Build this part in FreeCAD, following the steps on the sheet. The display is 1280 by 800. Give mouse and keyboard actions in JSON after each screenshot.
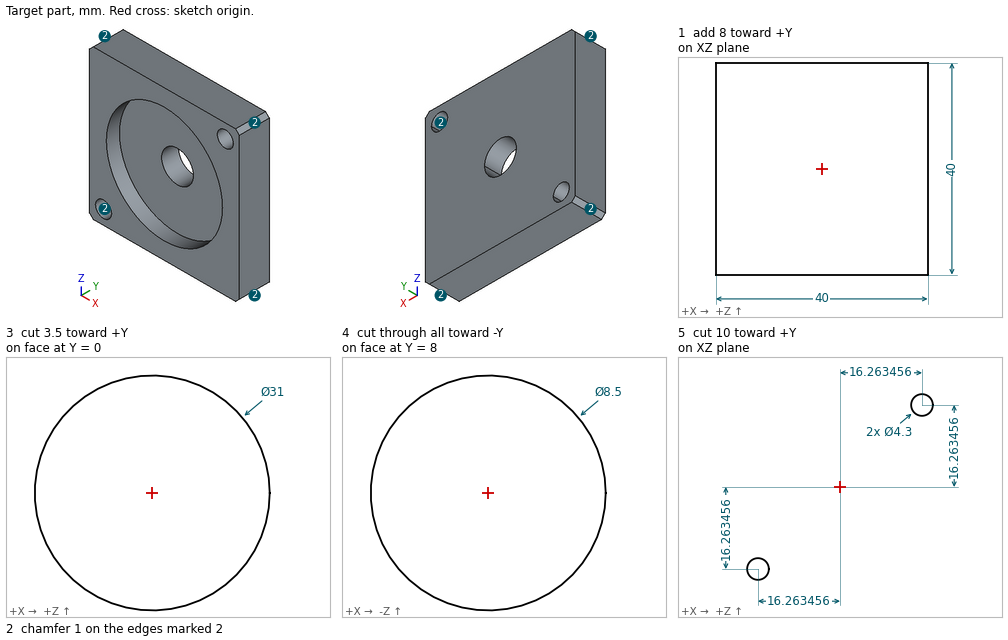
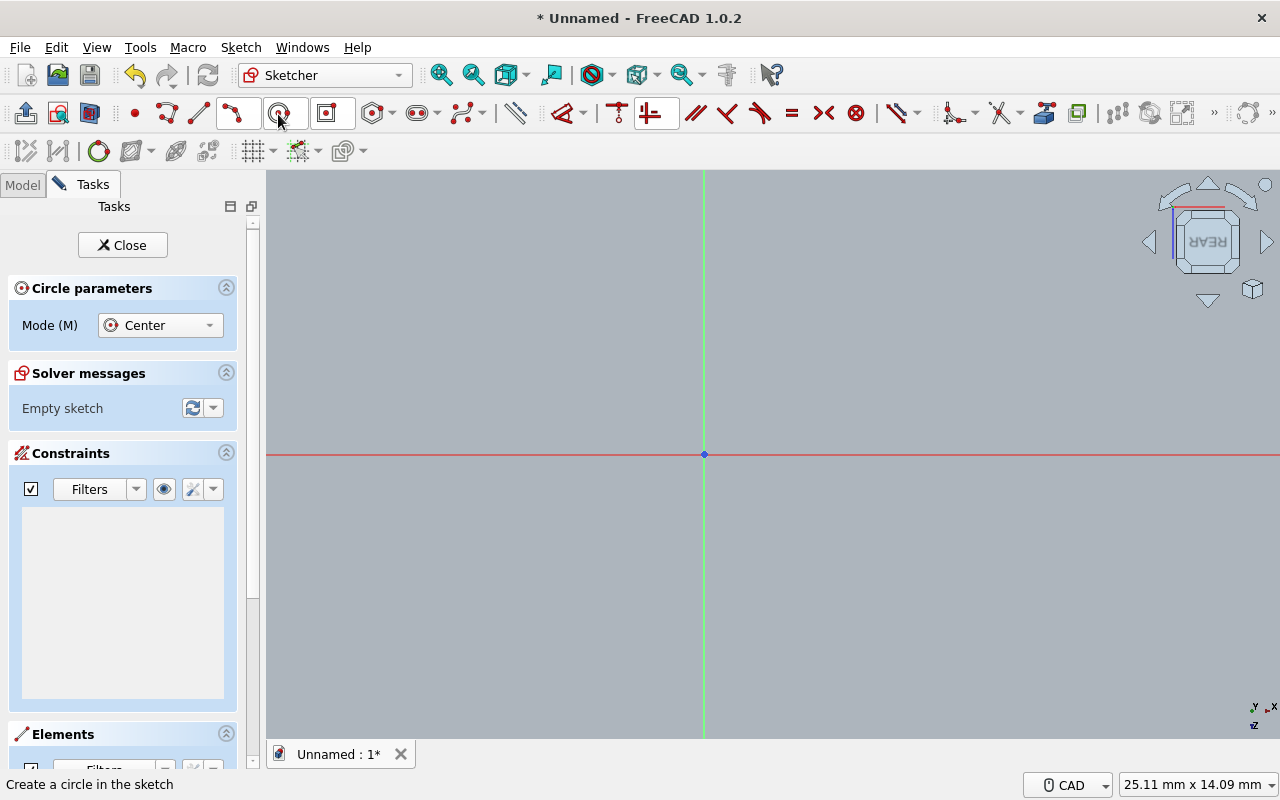
{"action": "left_click", "coordinate": [704, 454]}
{"action": "left_click", "coordinate": [826, 333]}
{"action": "key", "text": "Escape"}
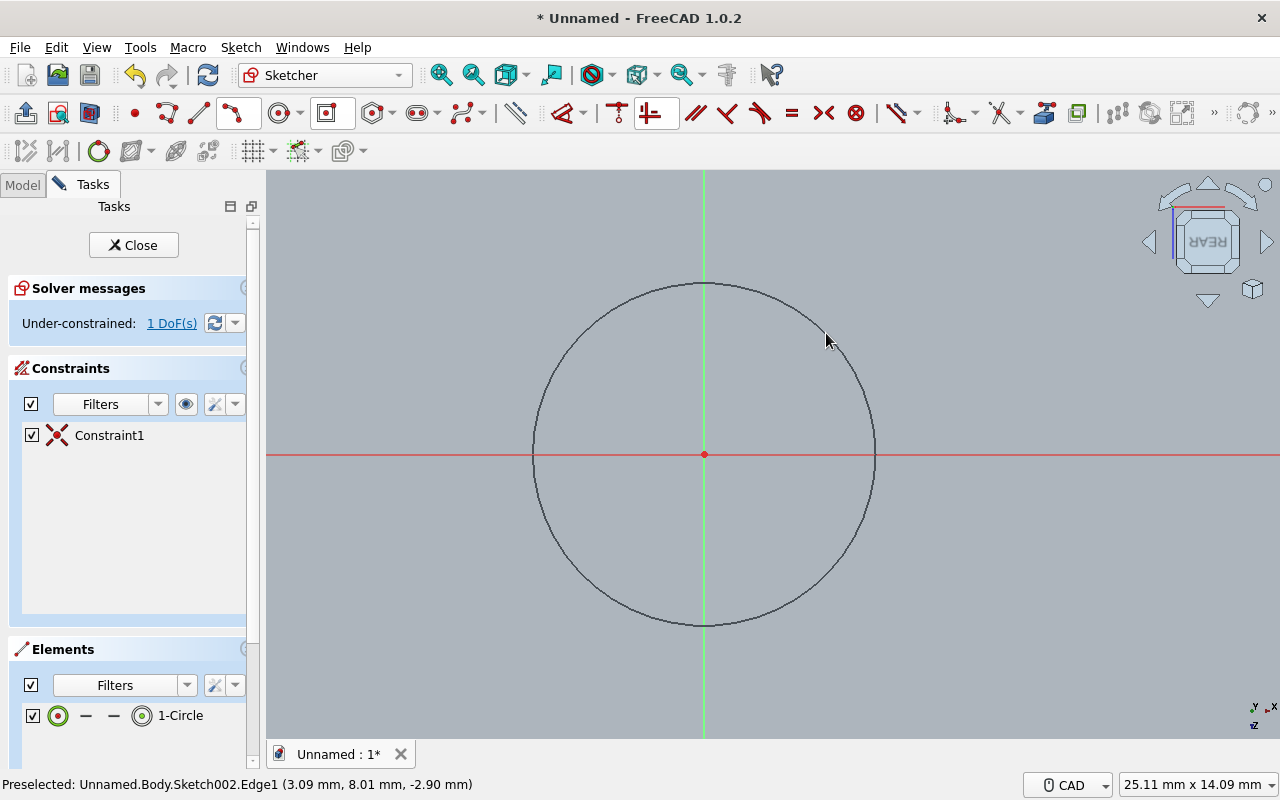
{"action": "left_click", "coordinate": [562, 114]}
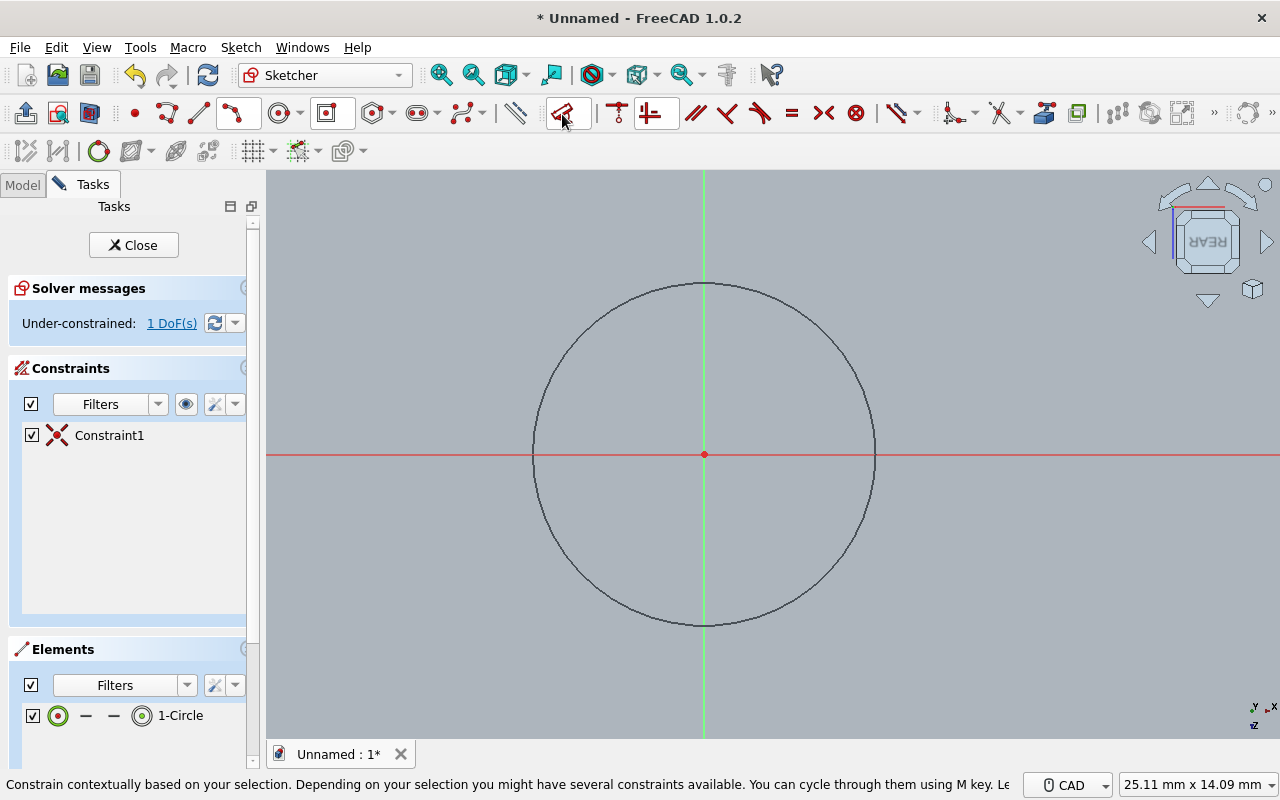
{"action": "left_click", "coordinate": [825, 333]}
{"action": "left_click", "coordinate": [848, 310]}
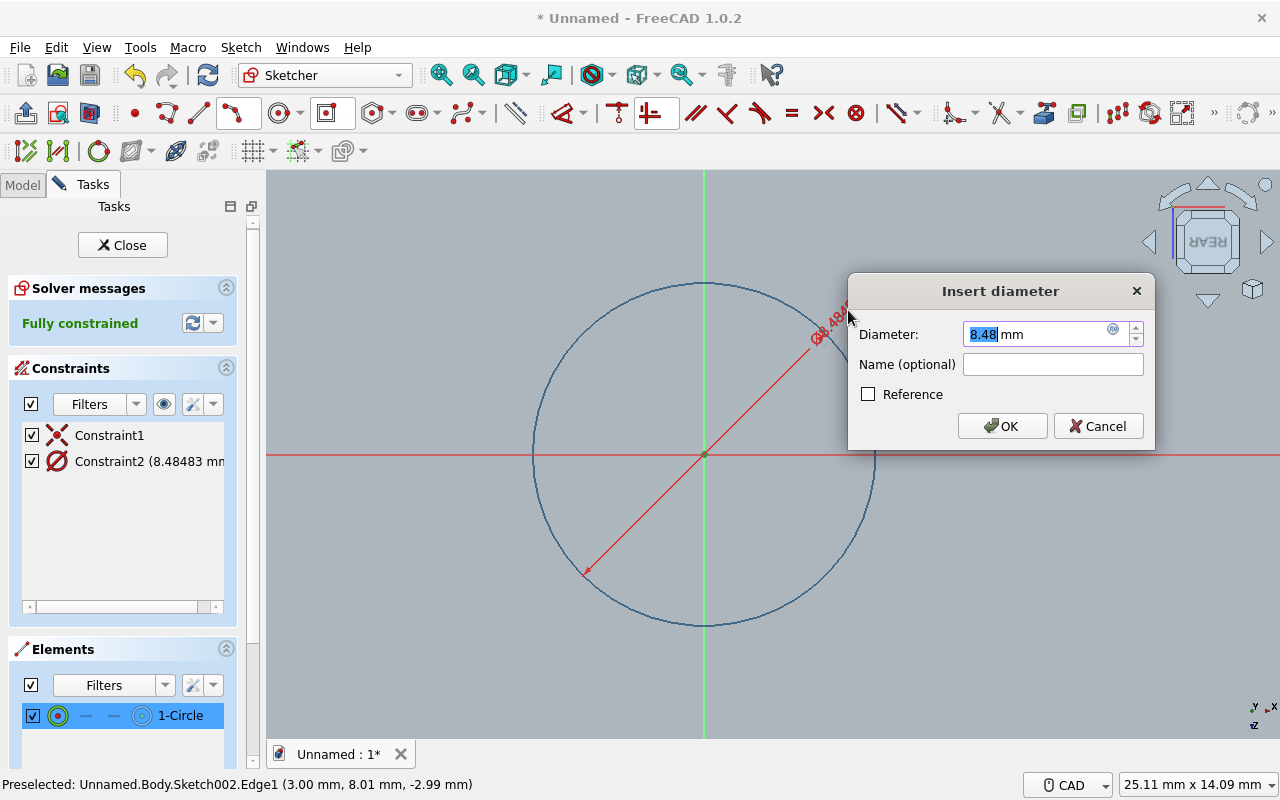
{"action": "type", "text": "8.5"}
{"action": "key", "text": "Return"}
{"action": "key", "text": "Escape"}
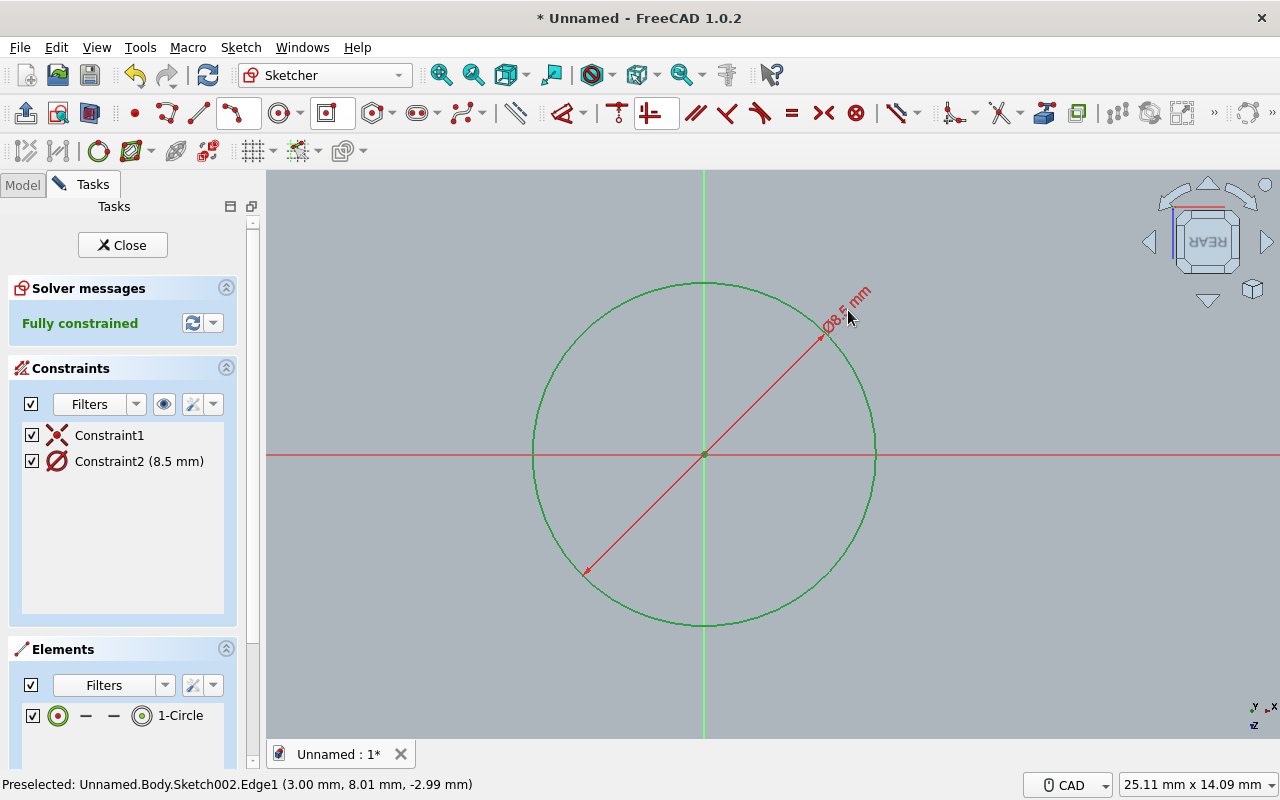
{"action": "left_click", "coordinate": [123, 245]}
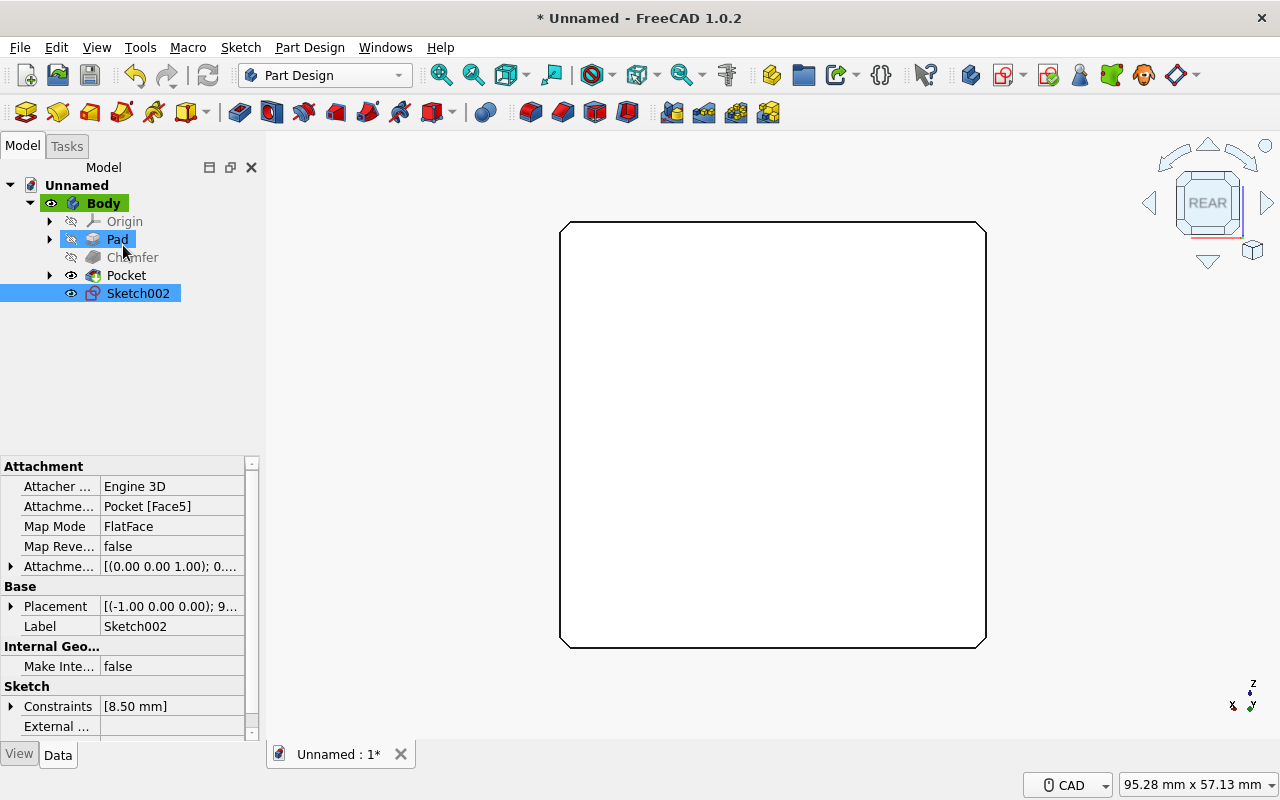
{"action": "left_click", "coordinate": [240, 112]}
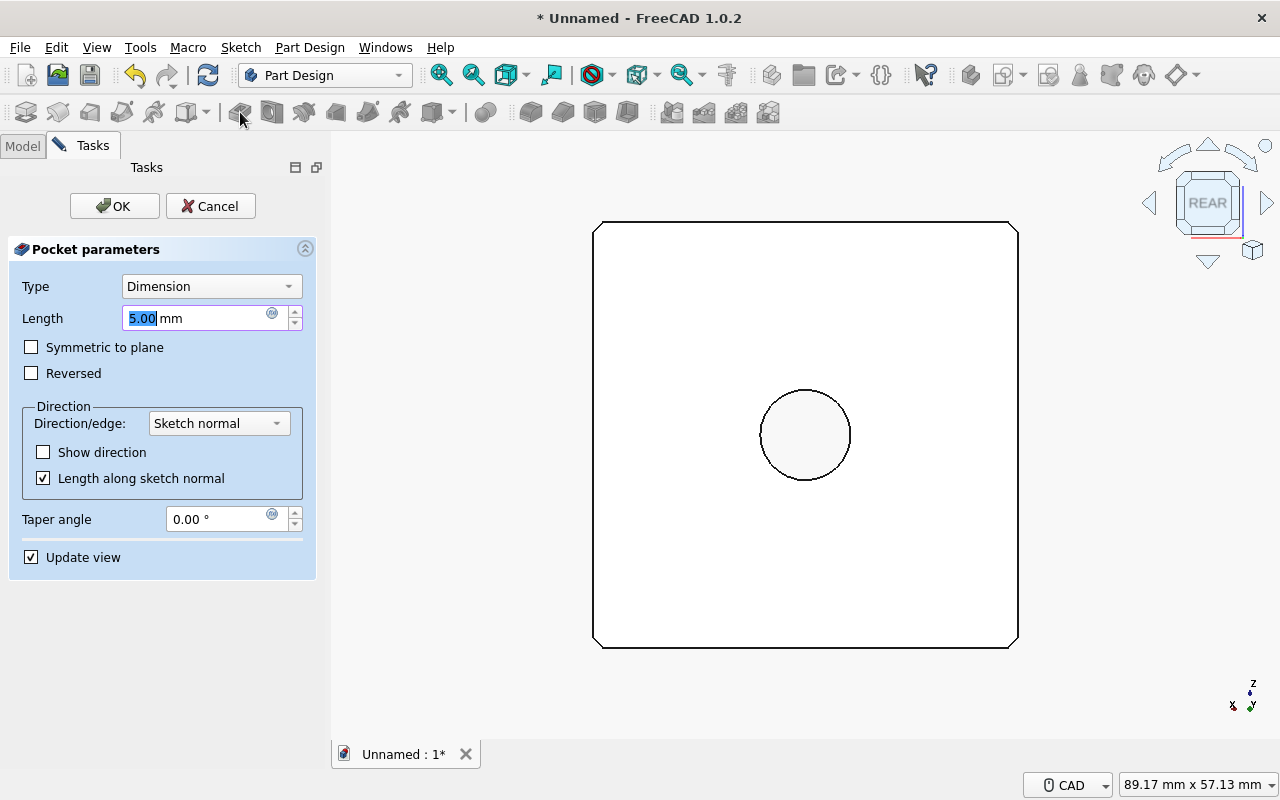
{"action": "left_click", "coordinate": [212, 286]}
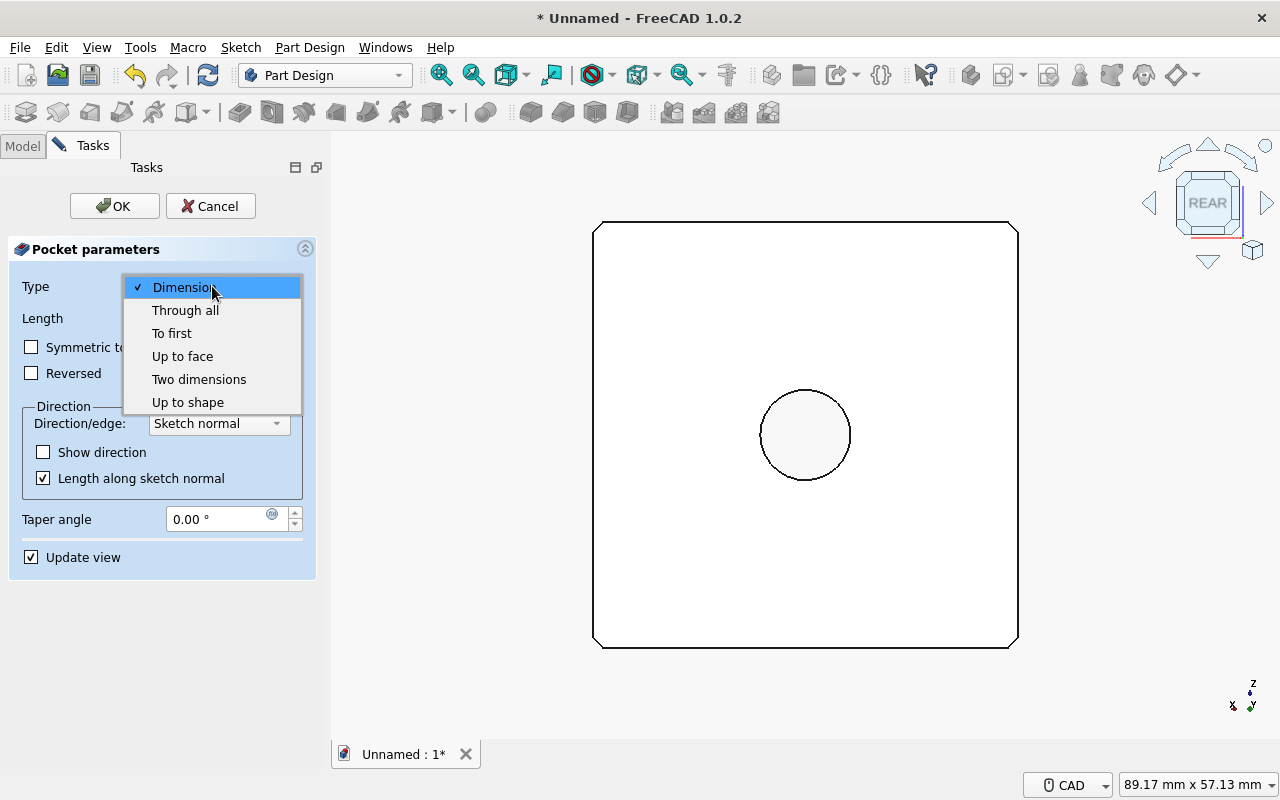
{"action": "left_click", "coordinate": [212, 310]}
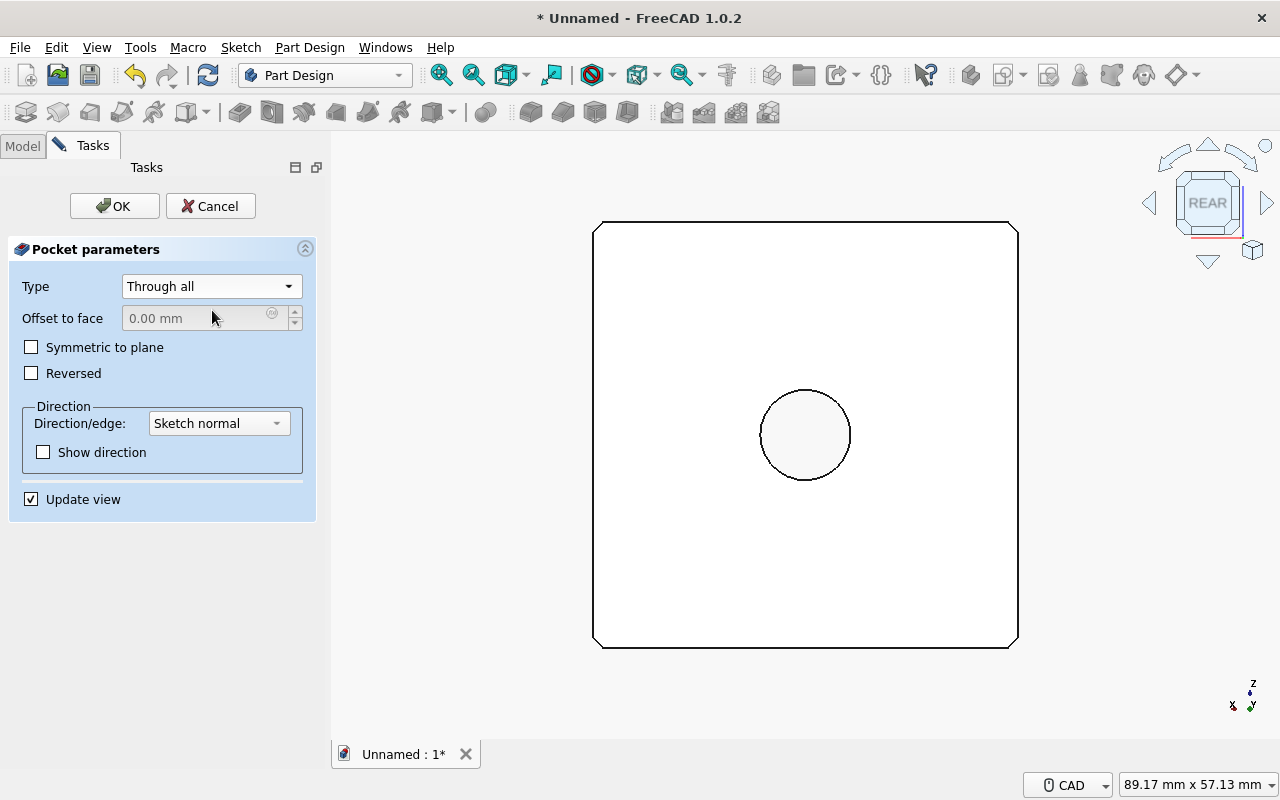
{"action": "left_click", "coordinate": [115, 206]}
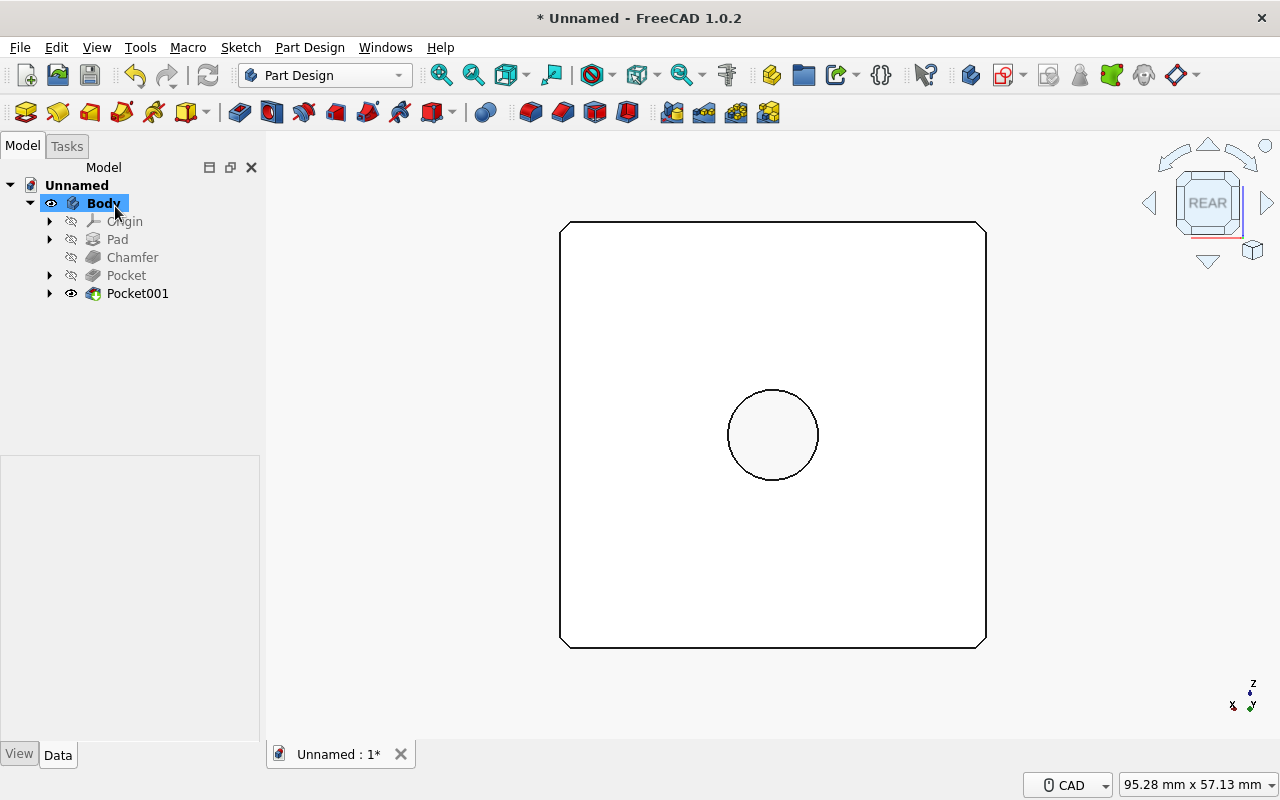
{"action": "left_click", "coordinate": [1004, 76]}